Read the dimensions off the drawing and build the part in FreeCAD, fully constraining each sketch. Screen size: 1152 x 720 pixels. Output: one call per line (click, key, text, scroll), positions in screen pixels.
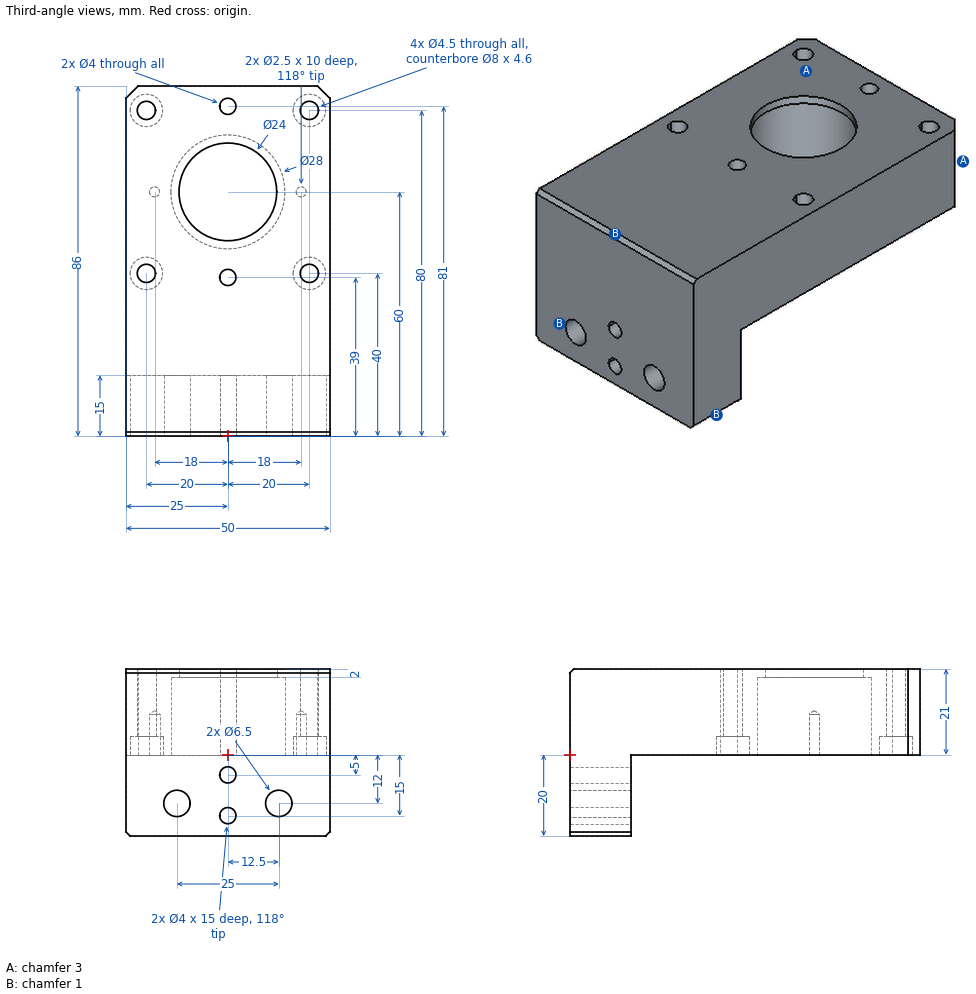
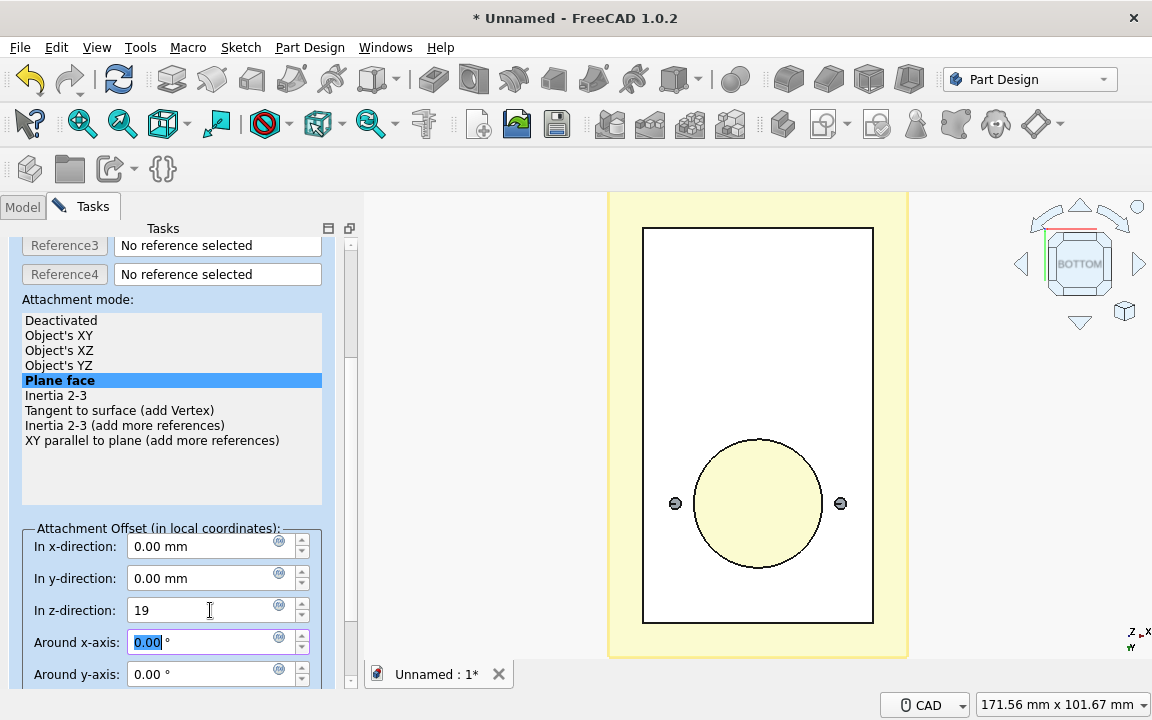
scroll(351, 463, up, 4)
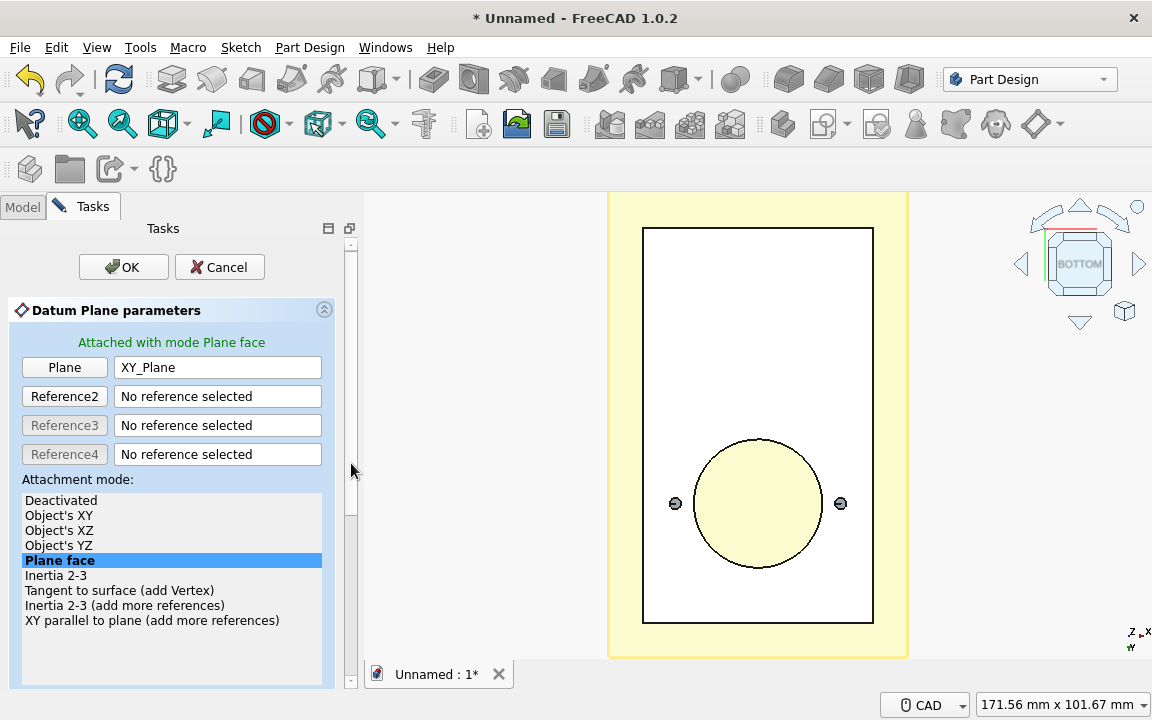
click(124, 267)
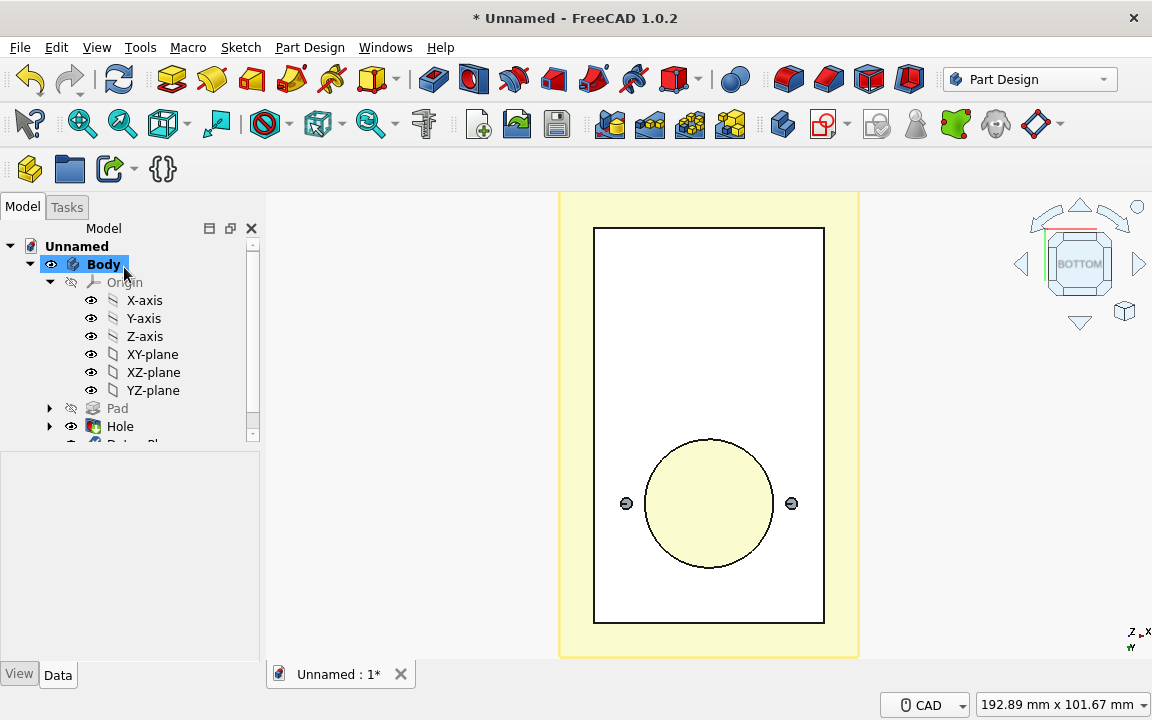
scroll(100, 332, down, 3)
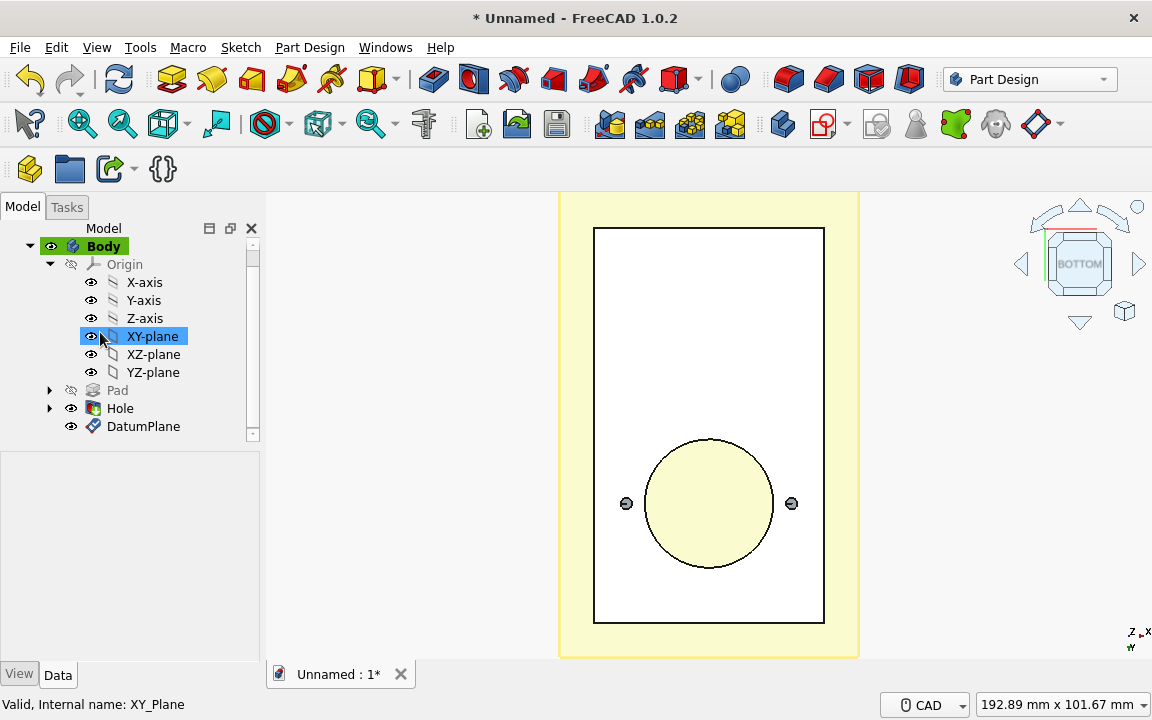
click(116, 426)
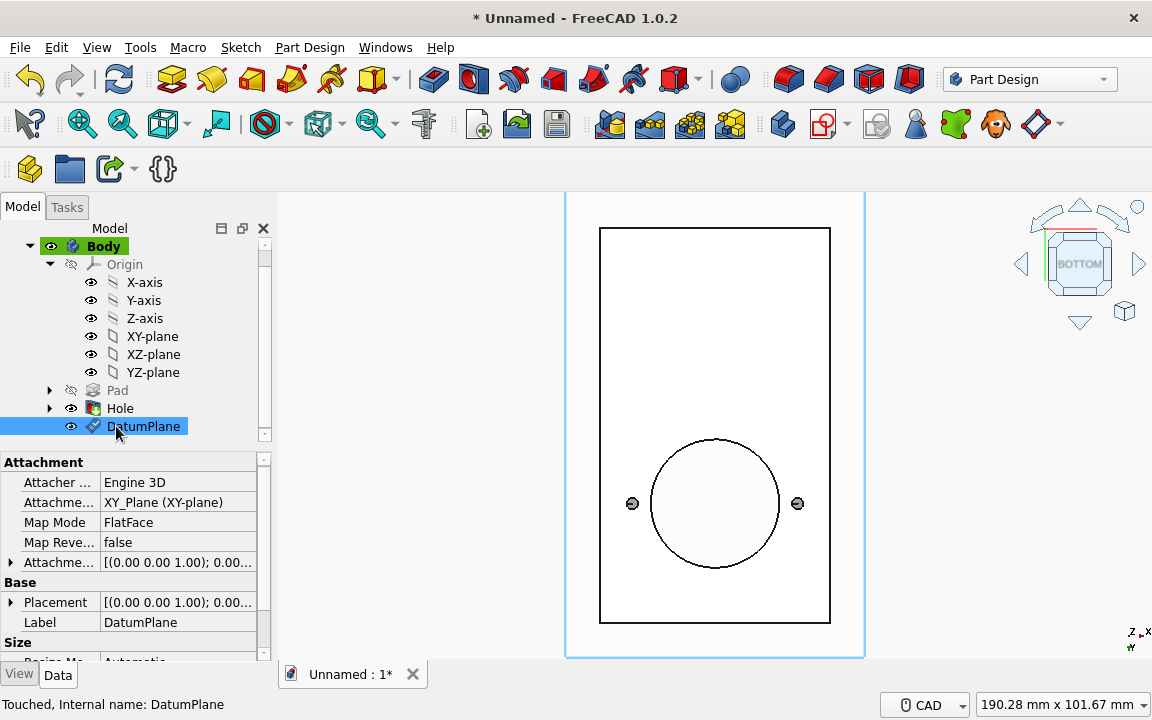
click(824, 124)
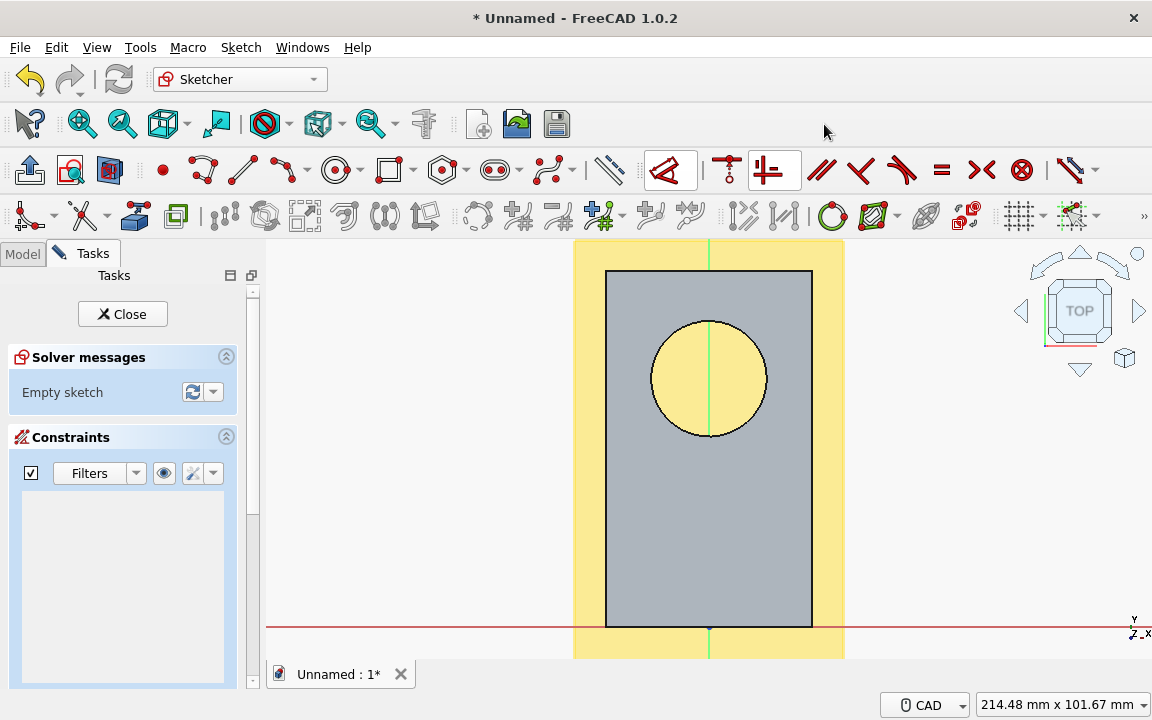
click(110, 170)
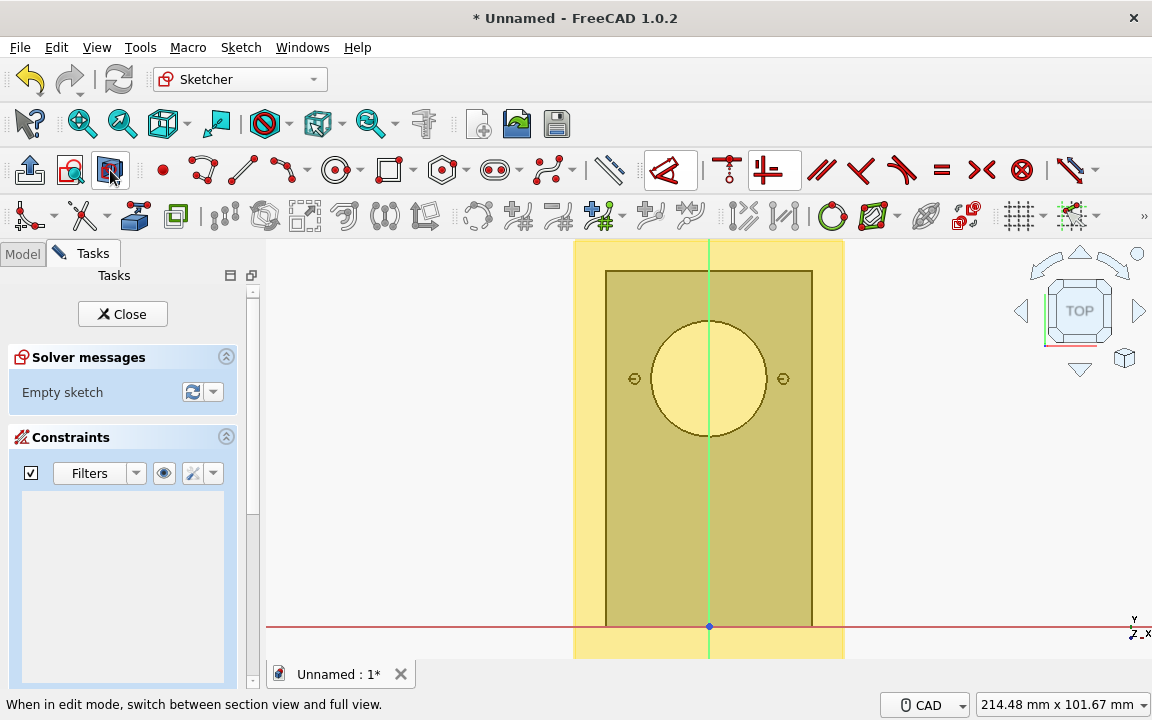
scroll(765, 321, up, 4)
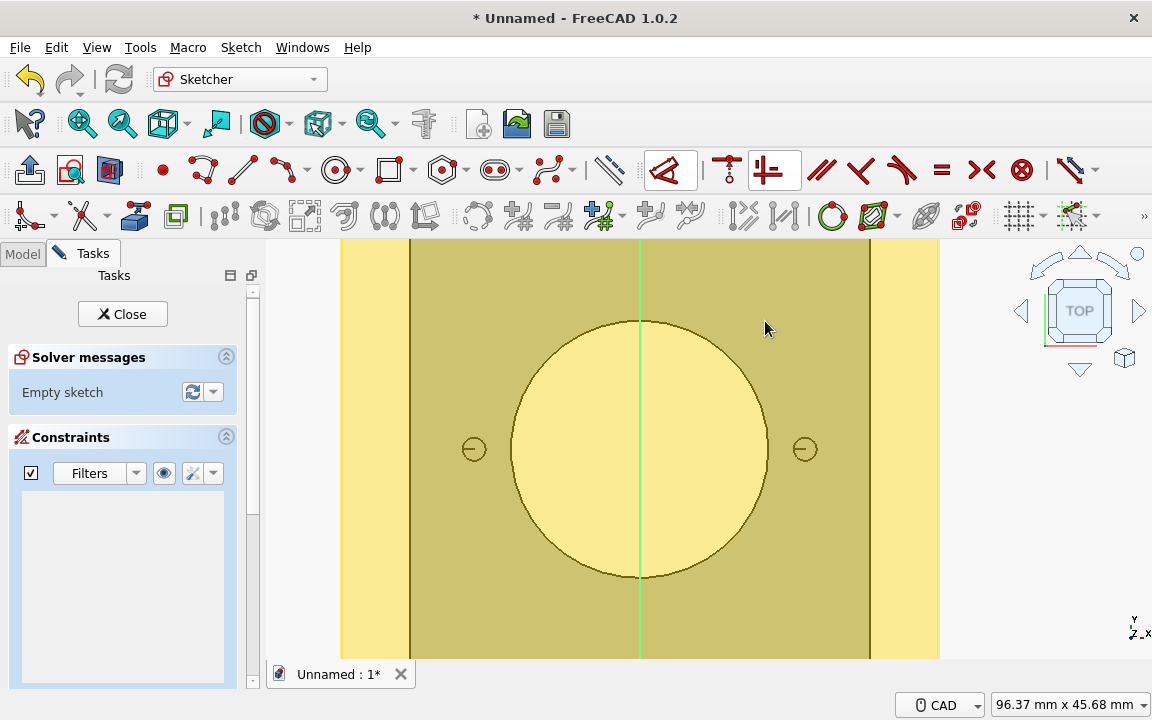
click(336, 170)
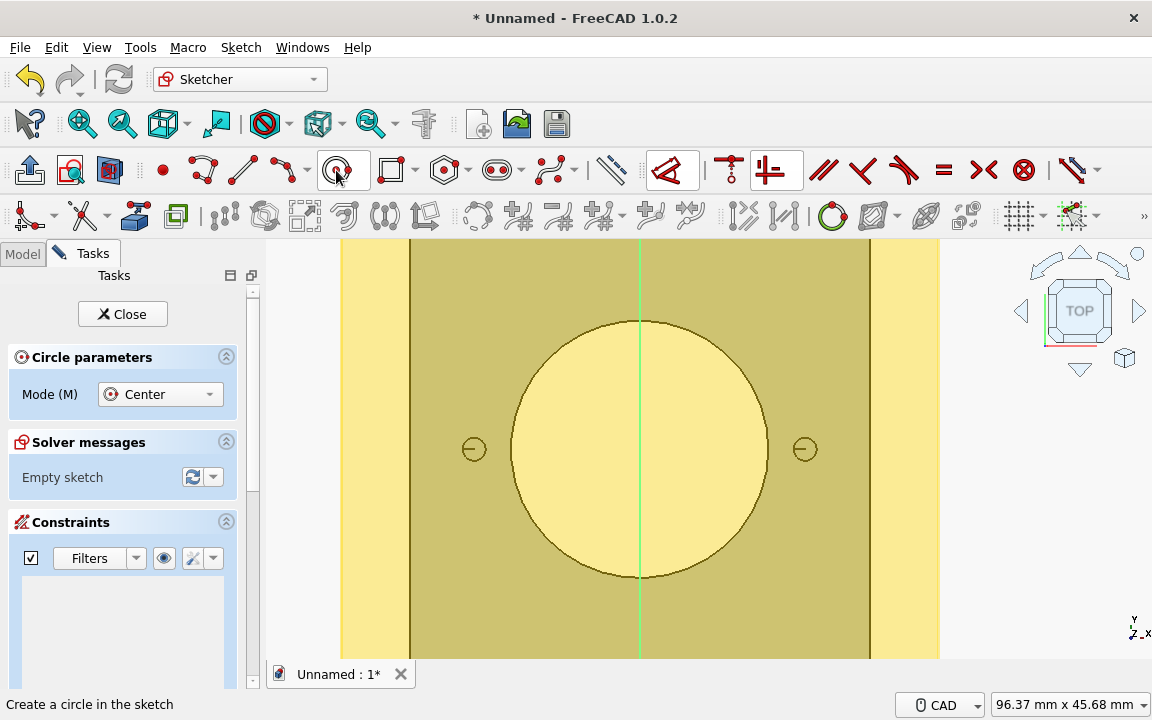
click(640, 449)
click(731, 358)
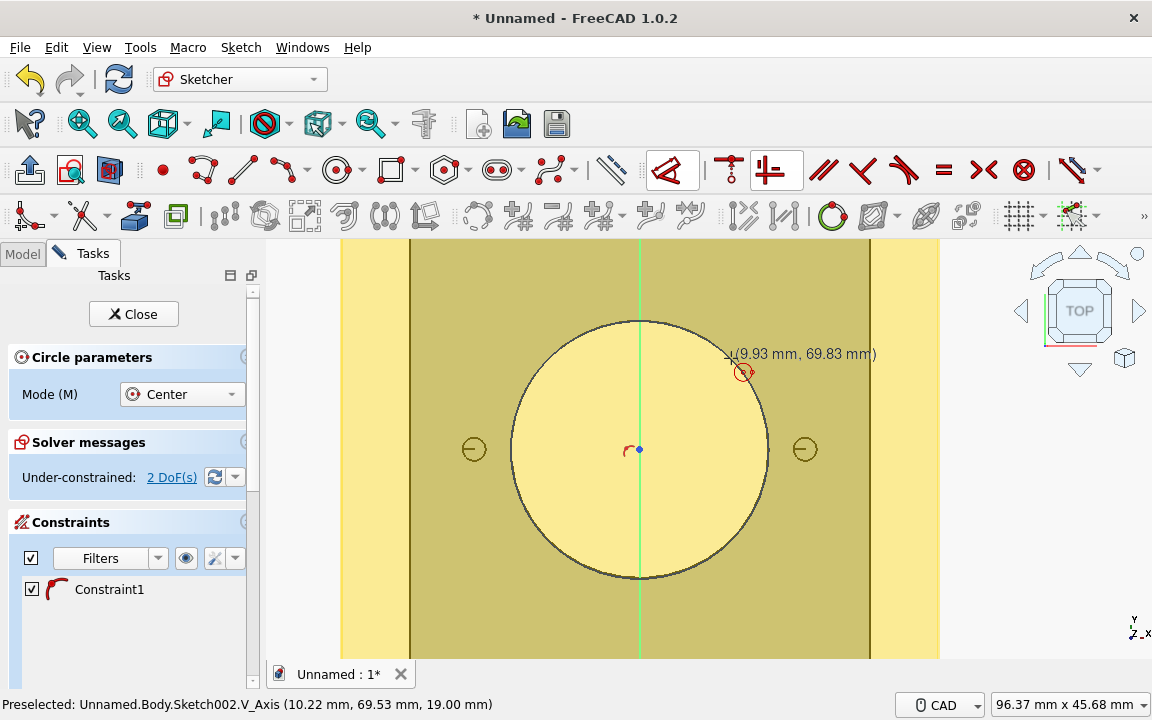
click(640, 450)
click(718, 371)
key(Escape)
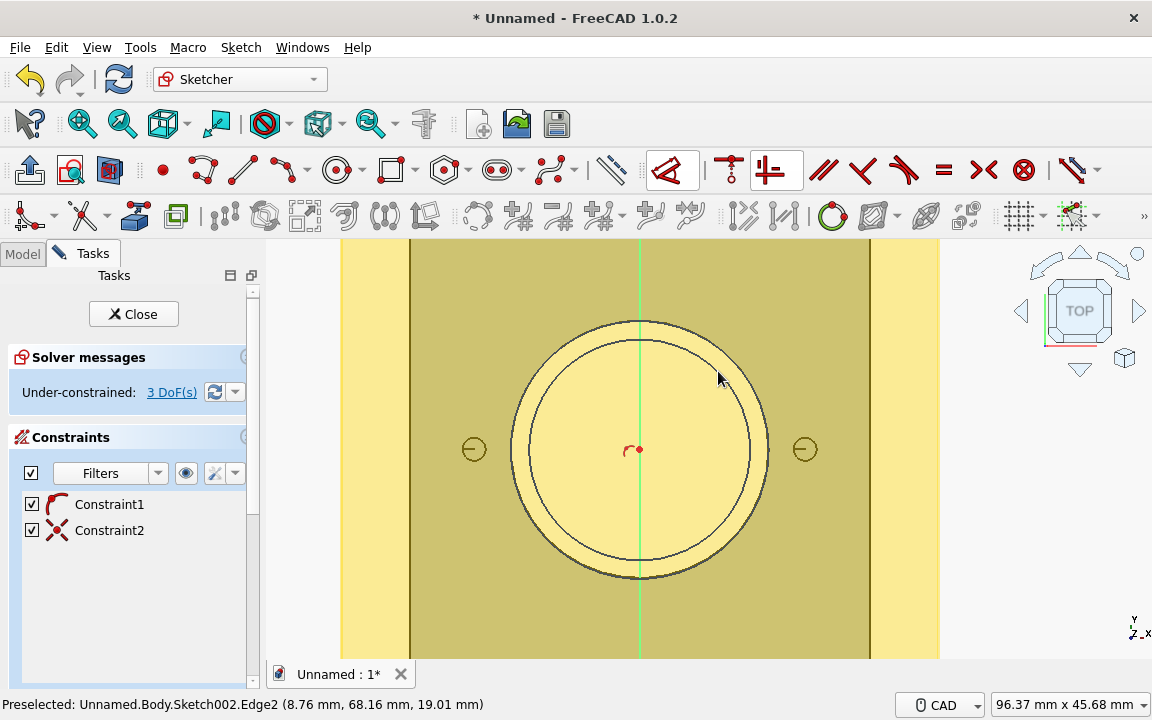
click(731, 359)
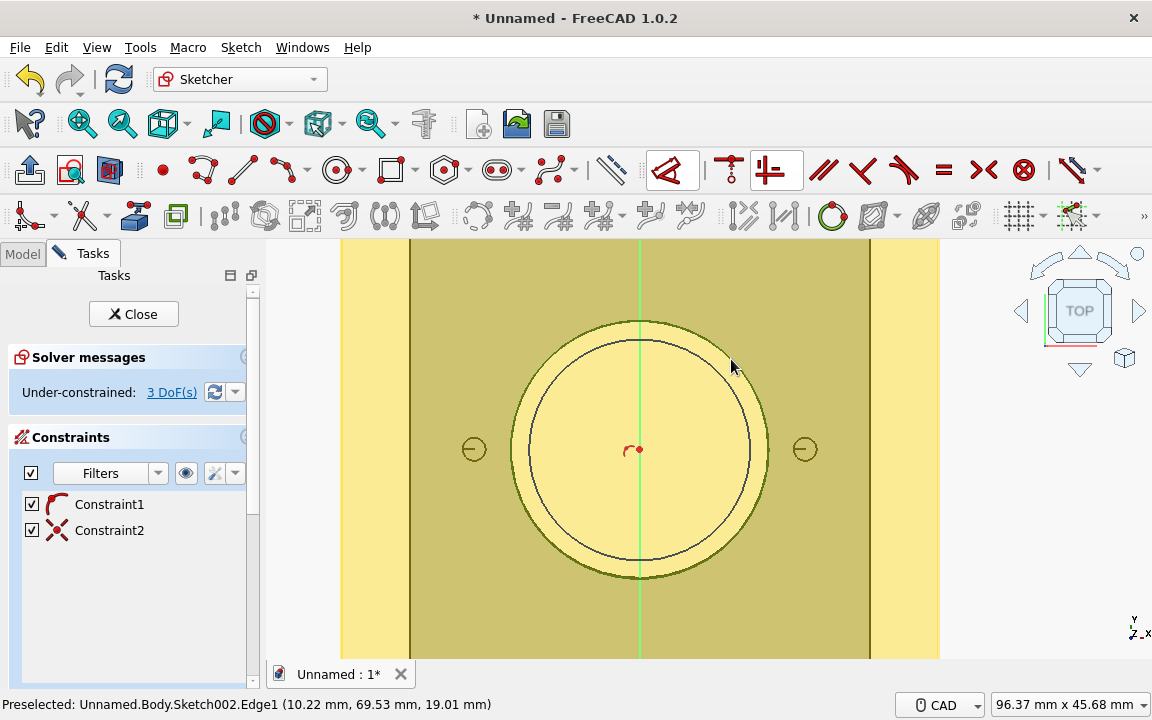
click(694, 170)